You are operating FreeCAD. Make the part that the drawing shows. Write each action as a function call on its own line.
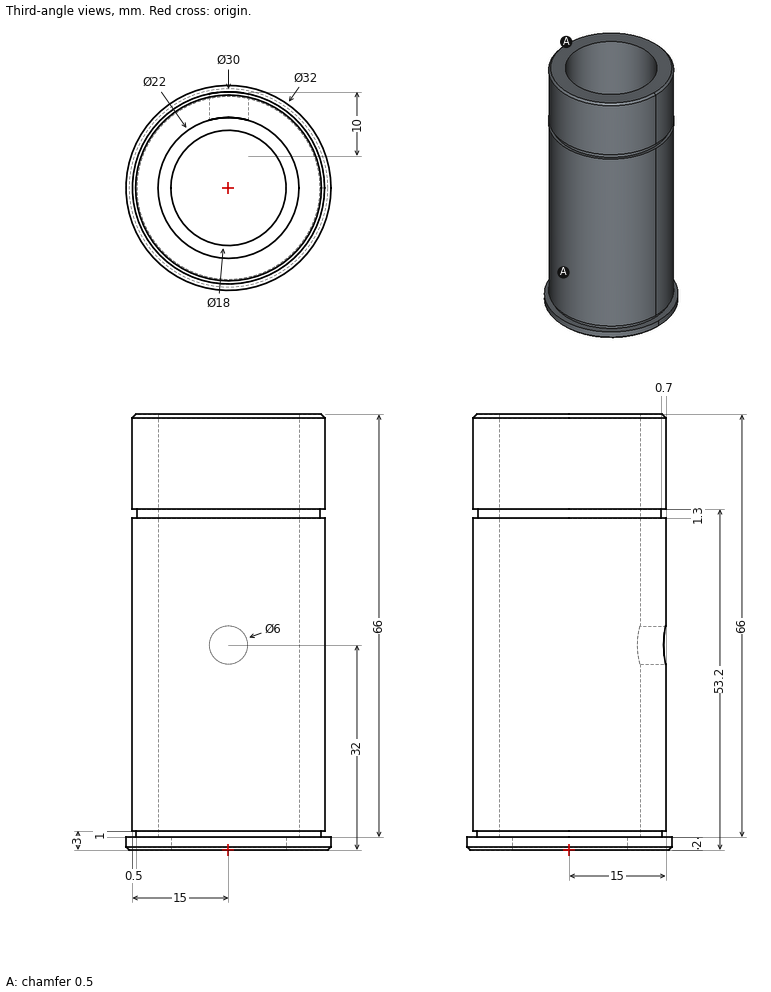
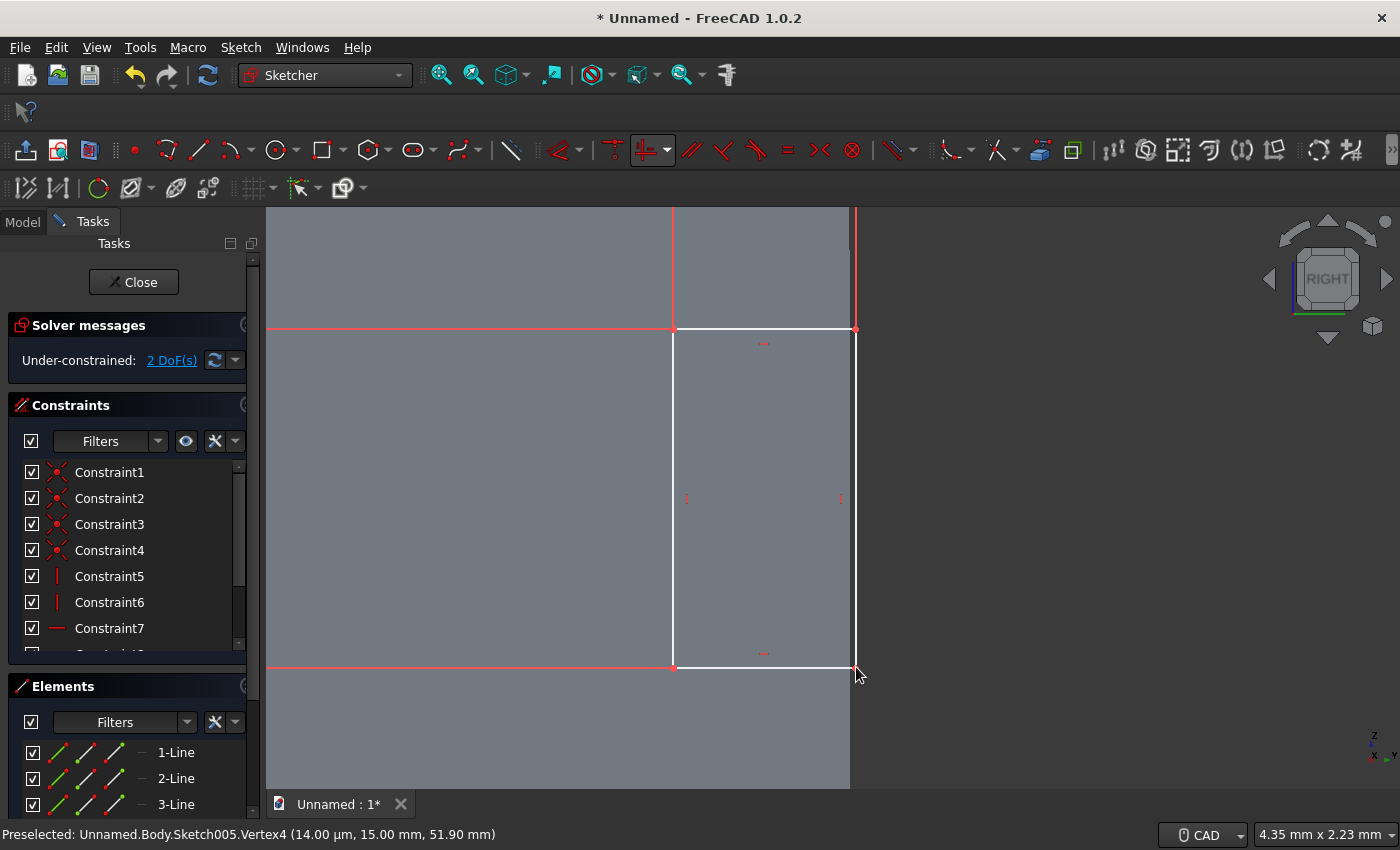
click(558, 150)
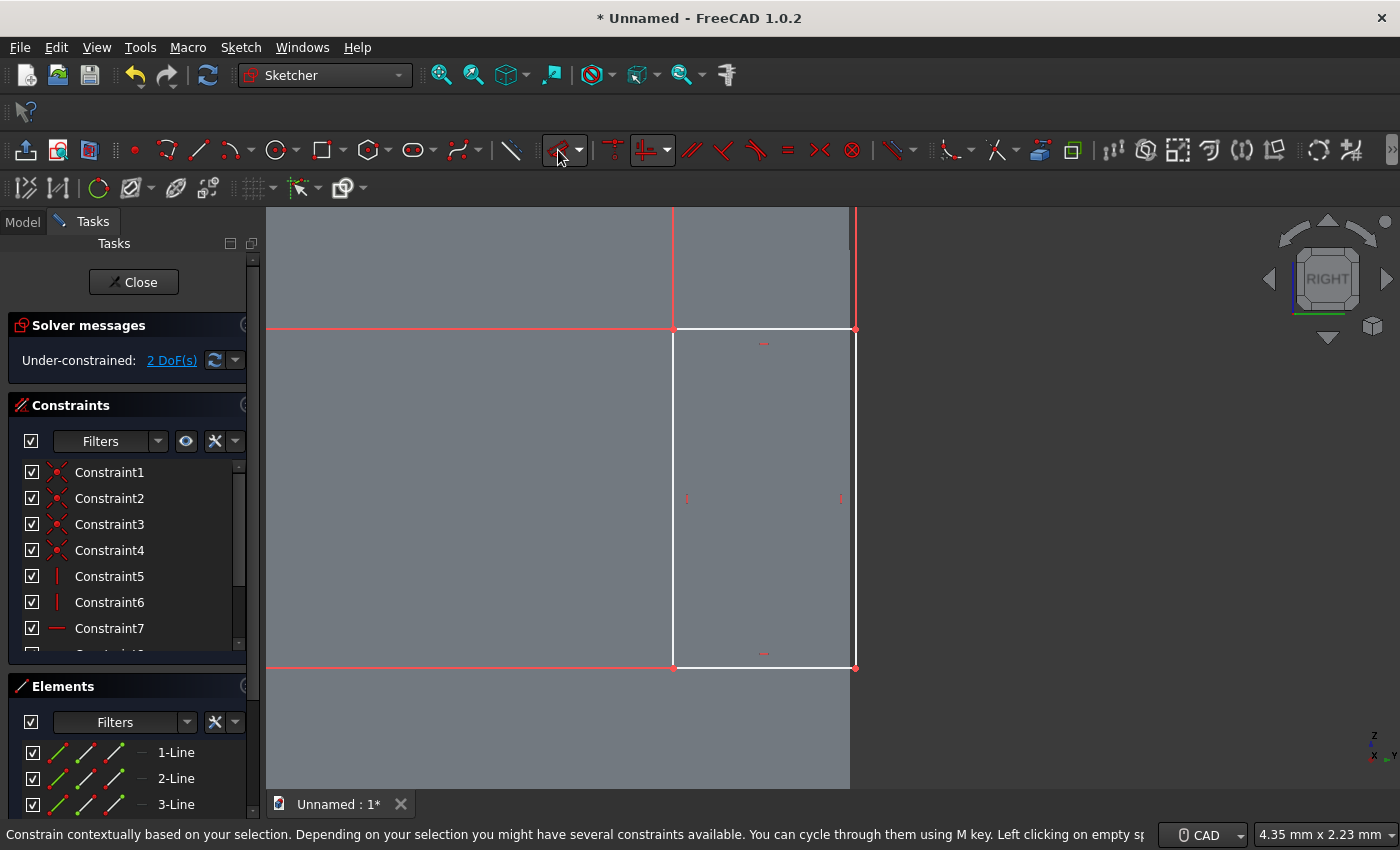
click(856, 668)
click(575, 634)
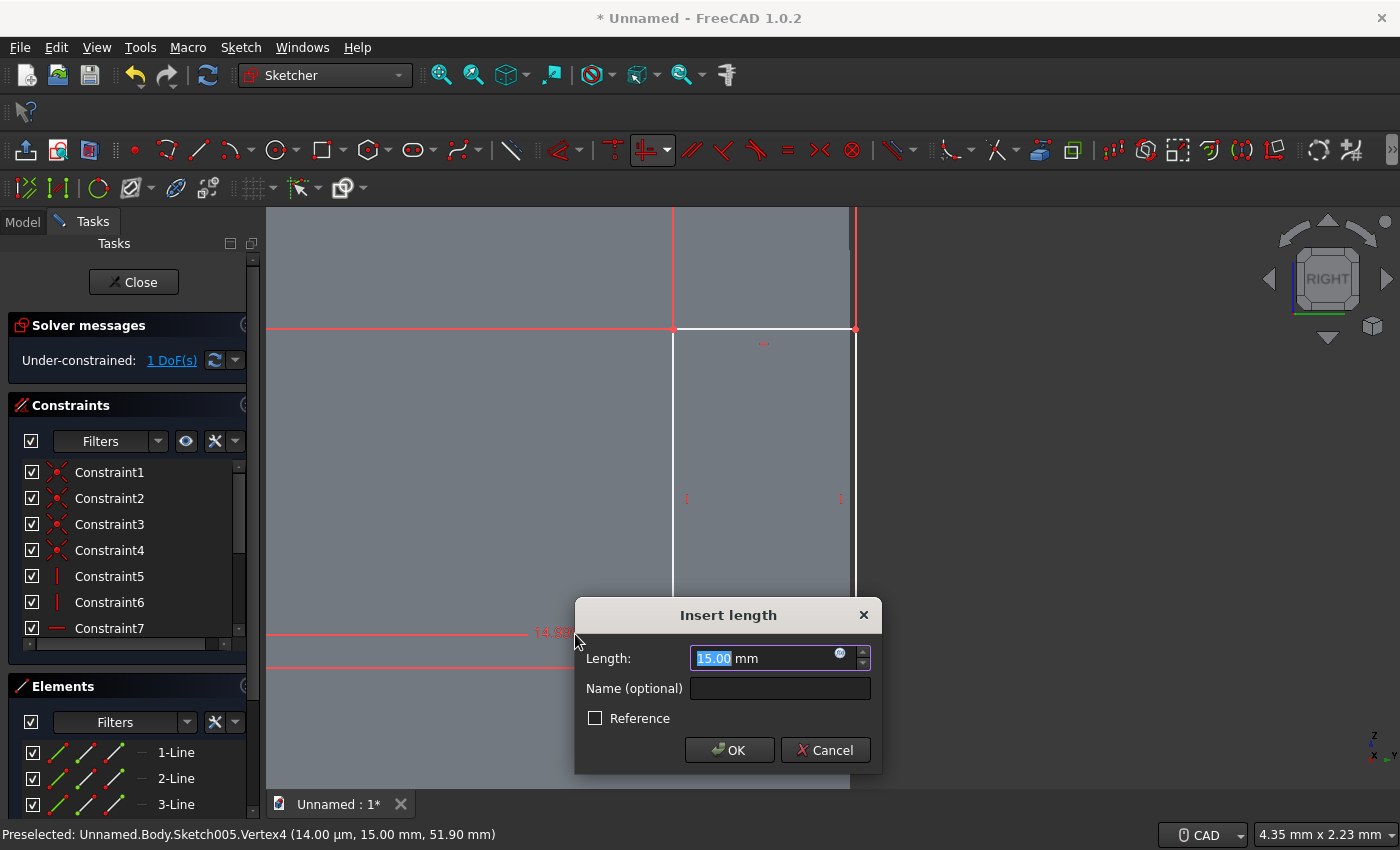
text(15)
key(Return)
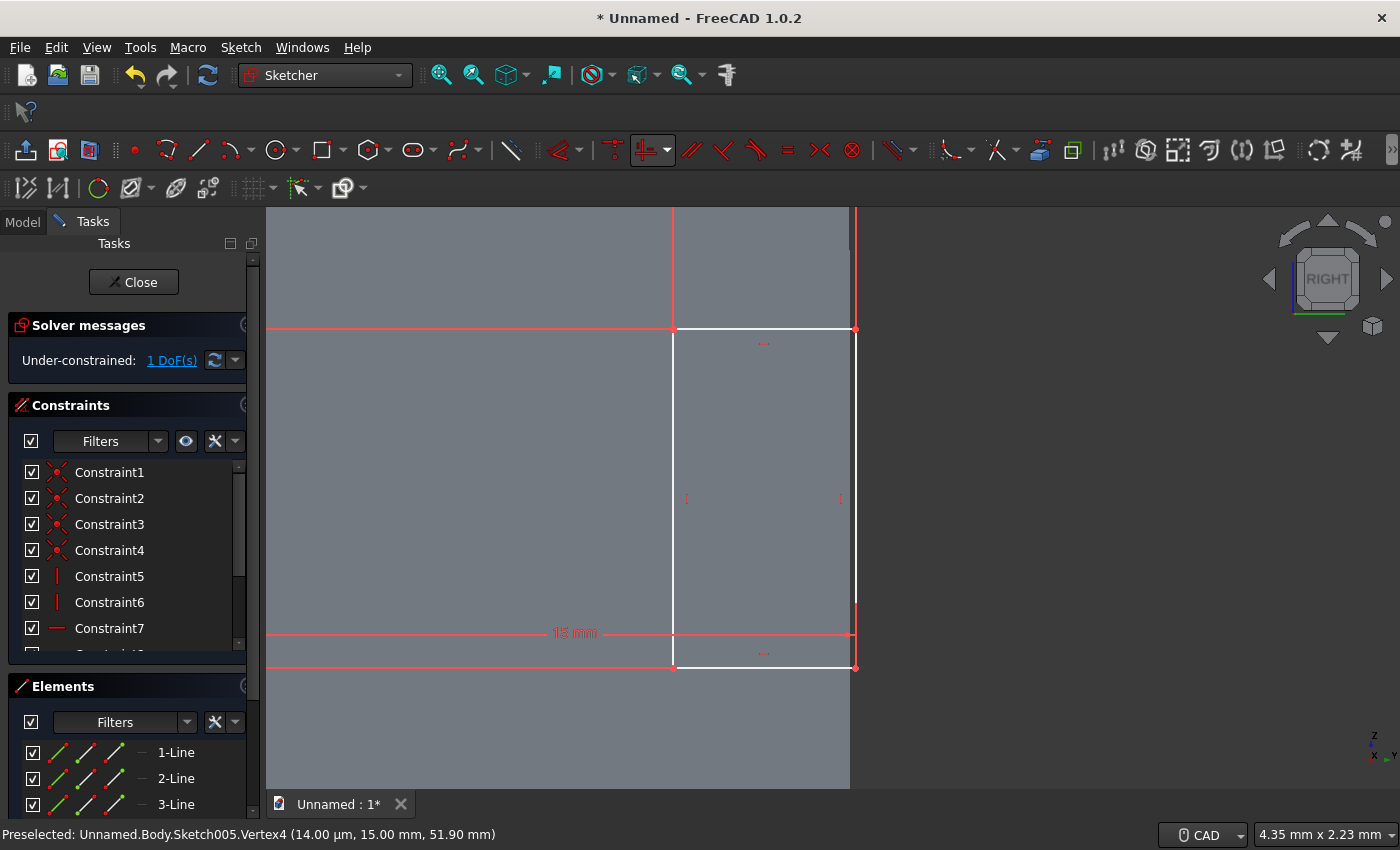
click(673, 329)
click(707, 545)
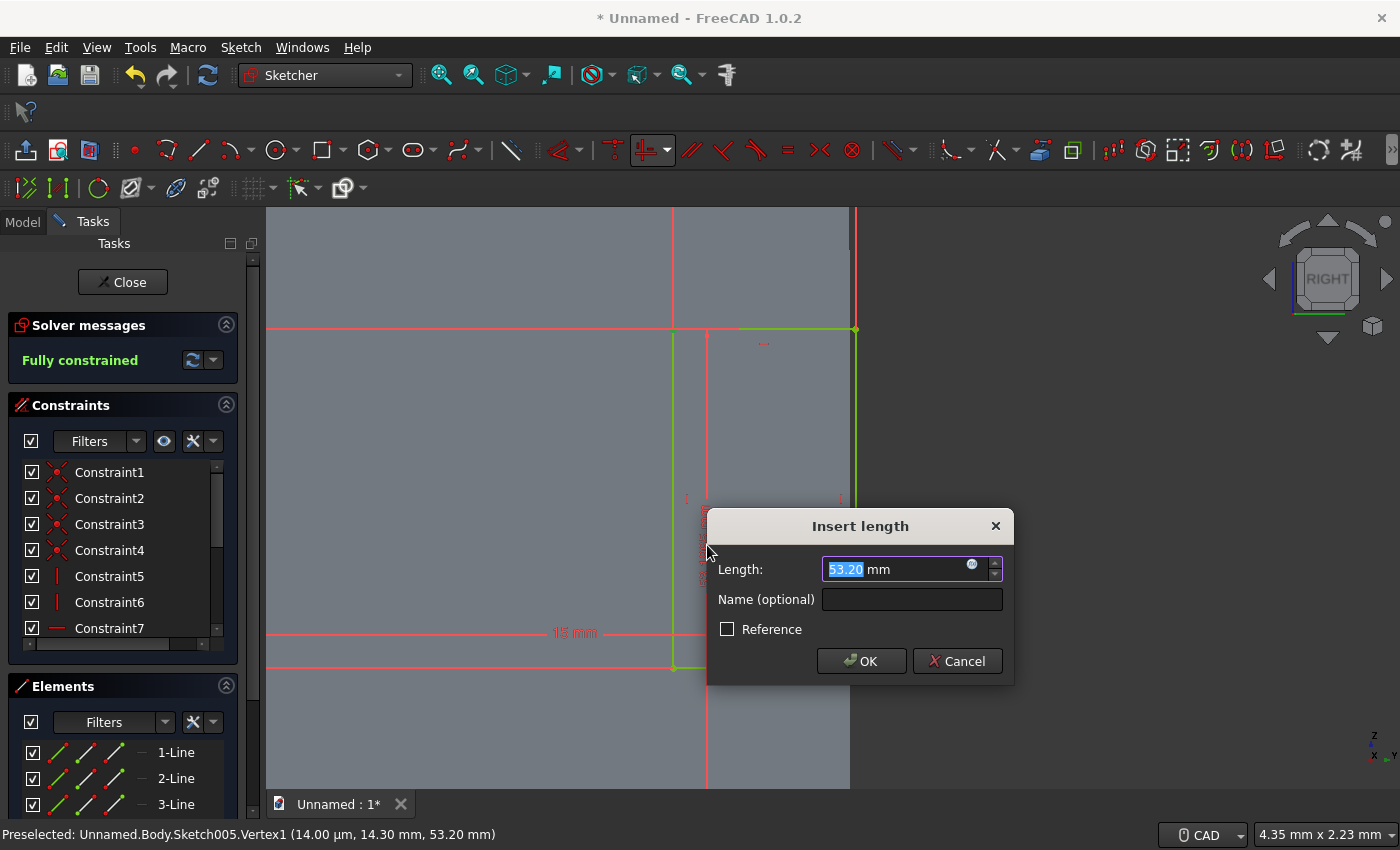
text(53.2)
key(Return)
key(Escape)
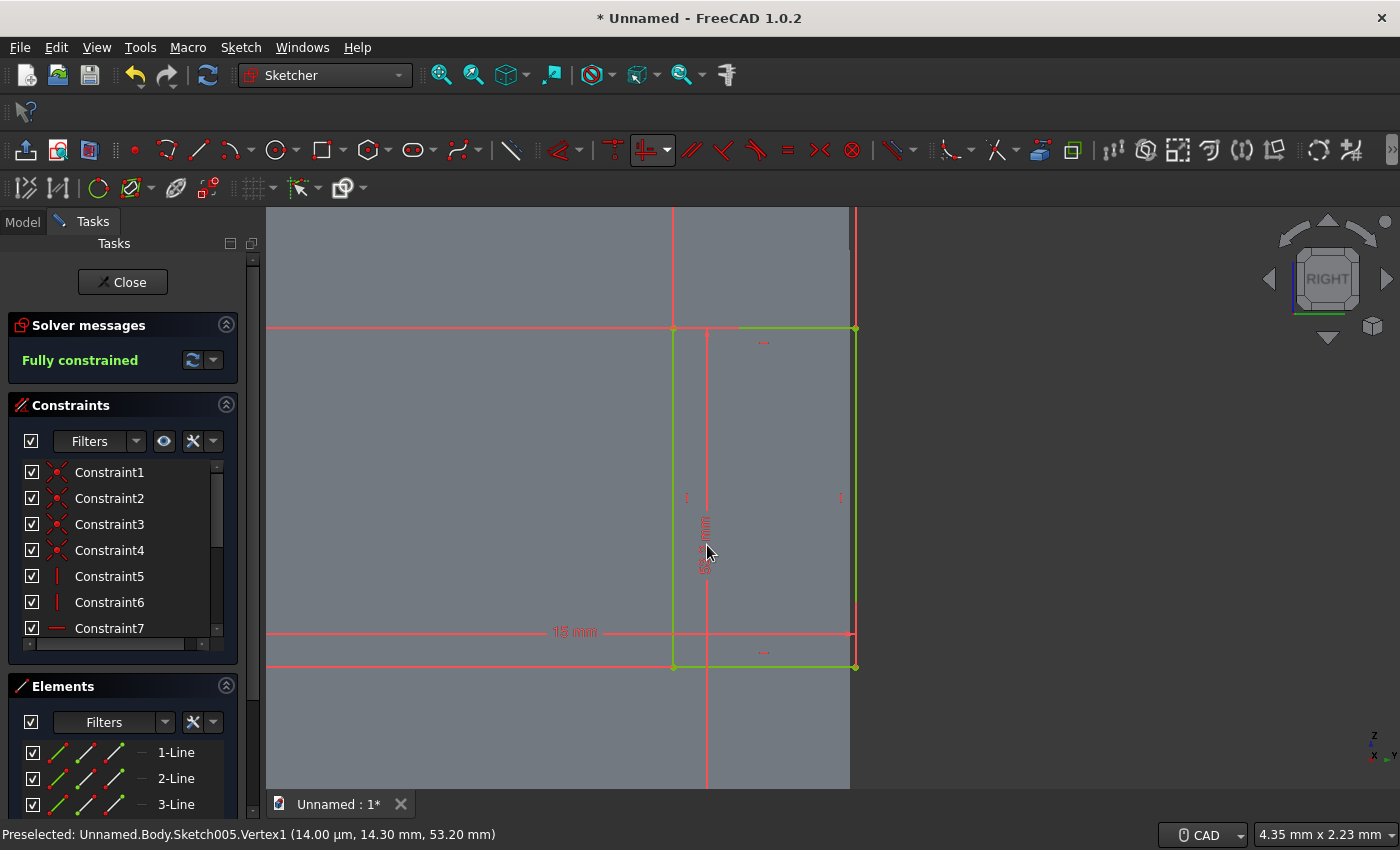
click(123, 282)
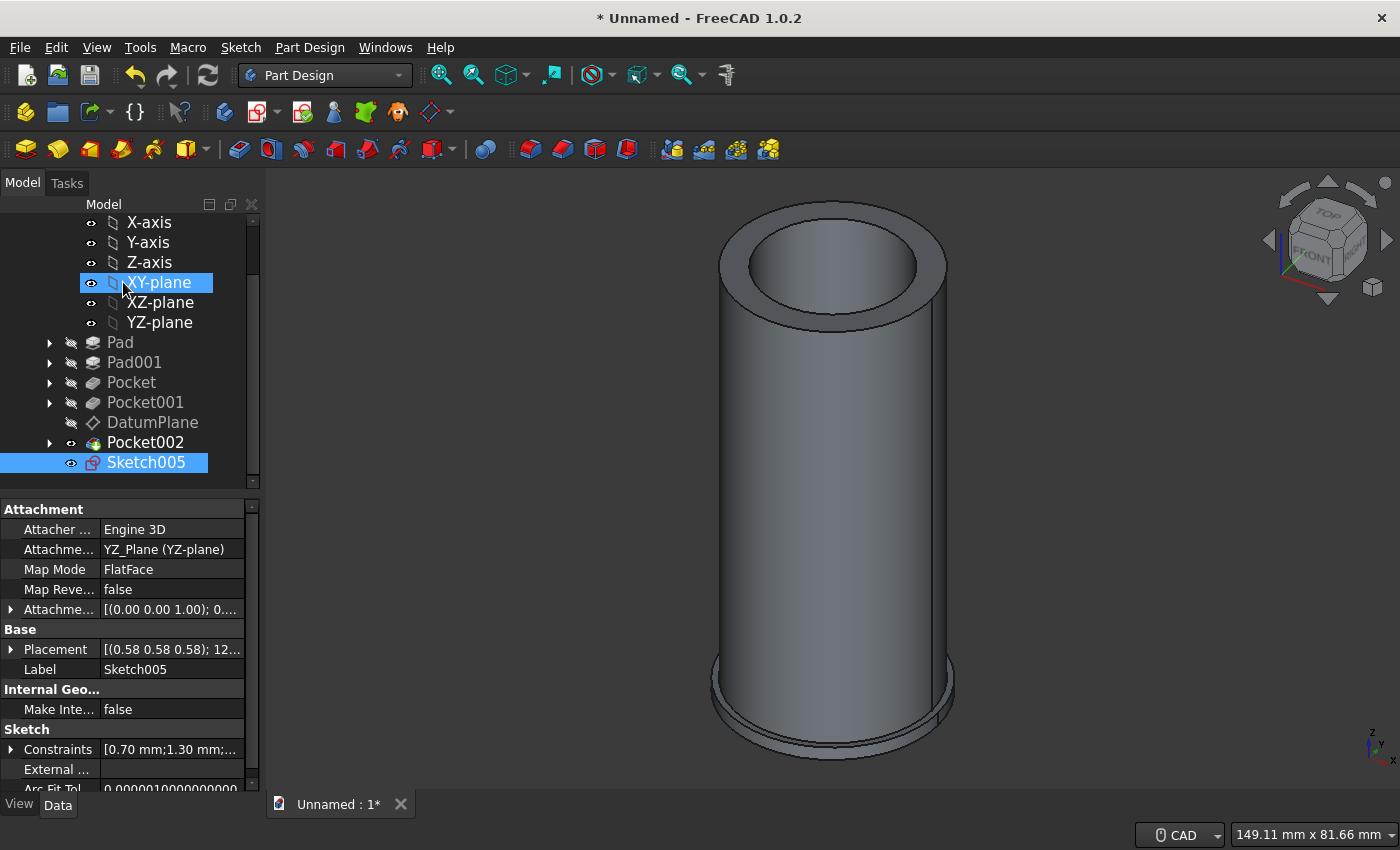
click(304, 150)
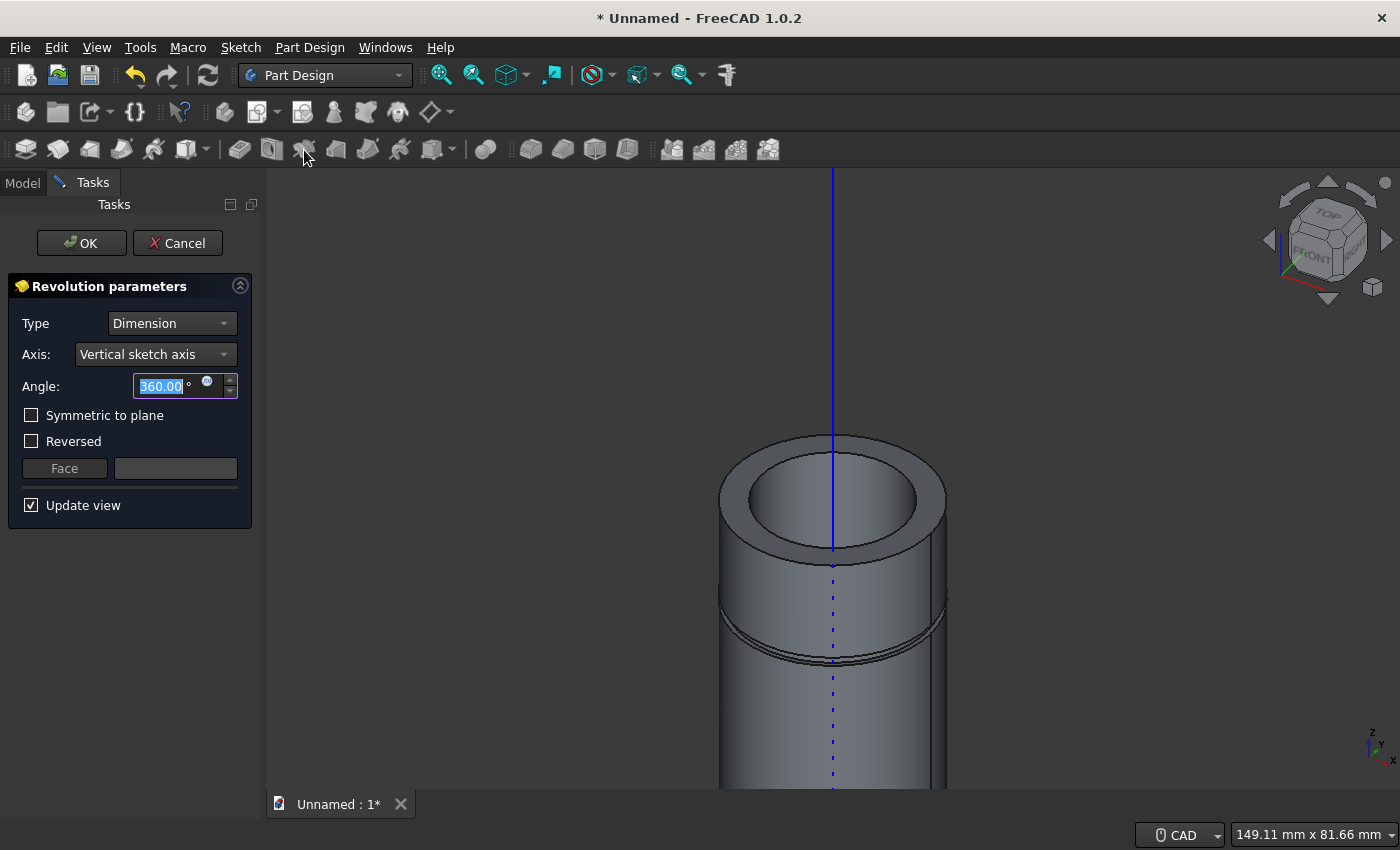
click(82, 243)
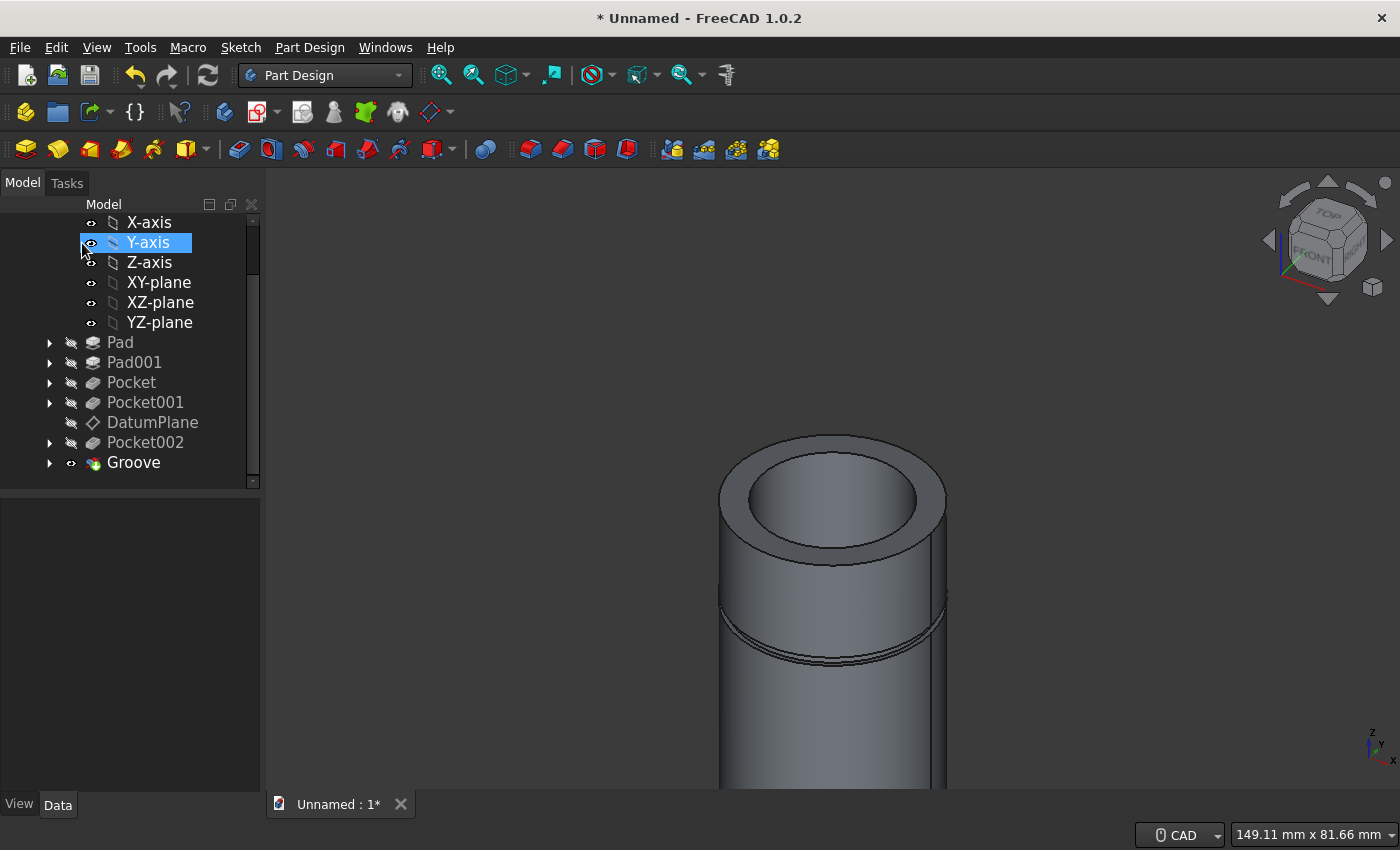
click(442, 76)